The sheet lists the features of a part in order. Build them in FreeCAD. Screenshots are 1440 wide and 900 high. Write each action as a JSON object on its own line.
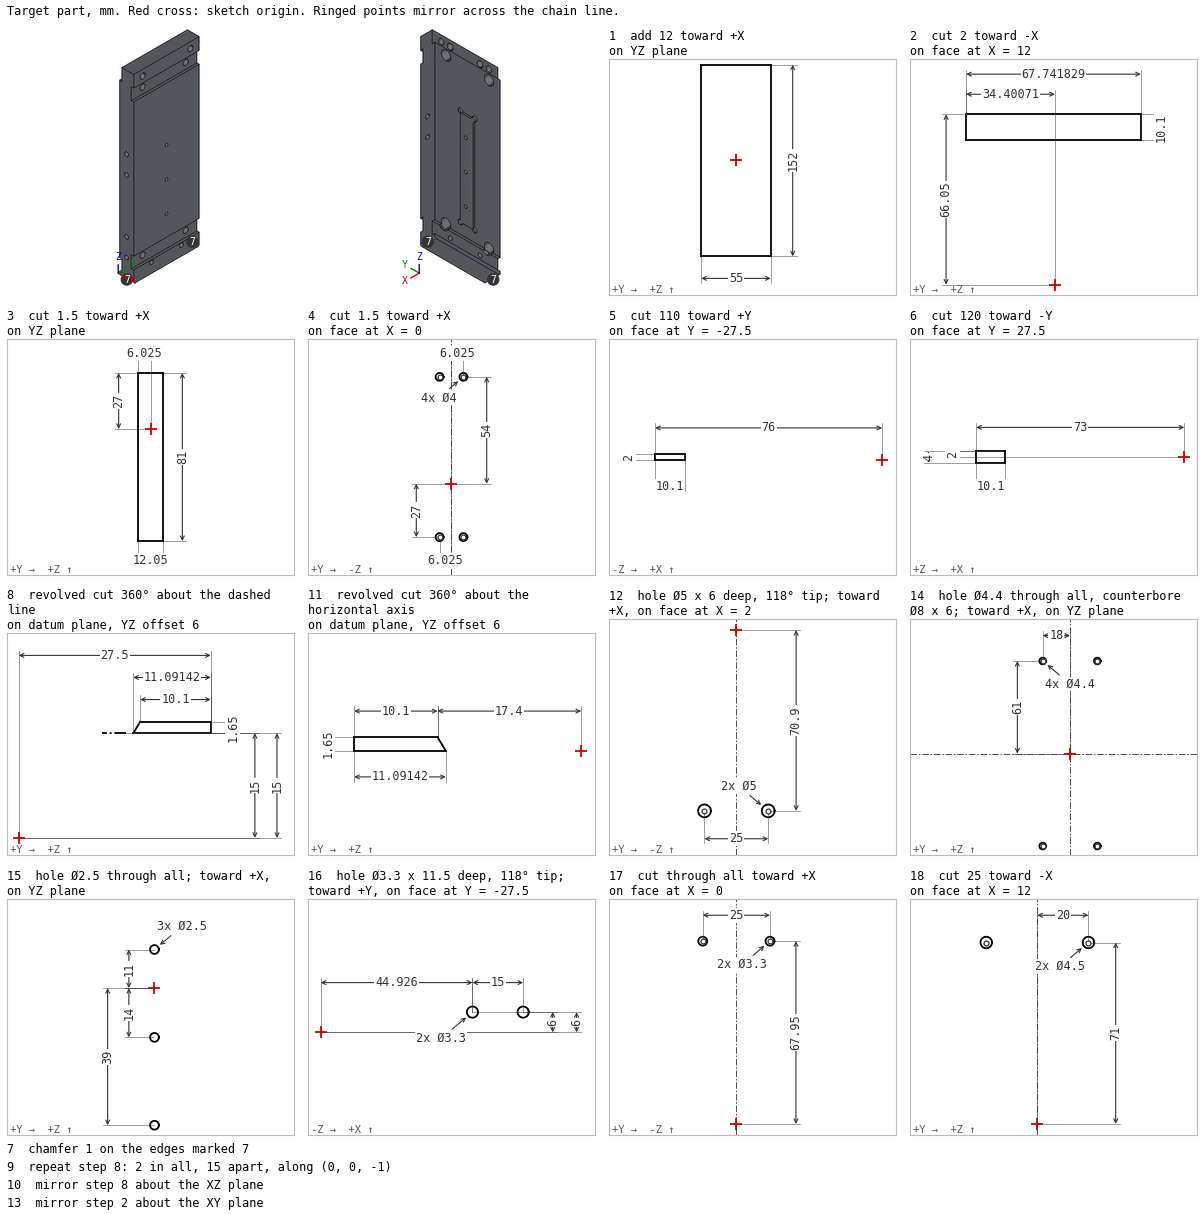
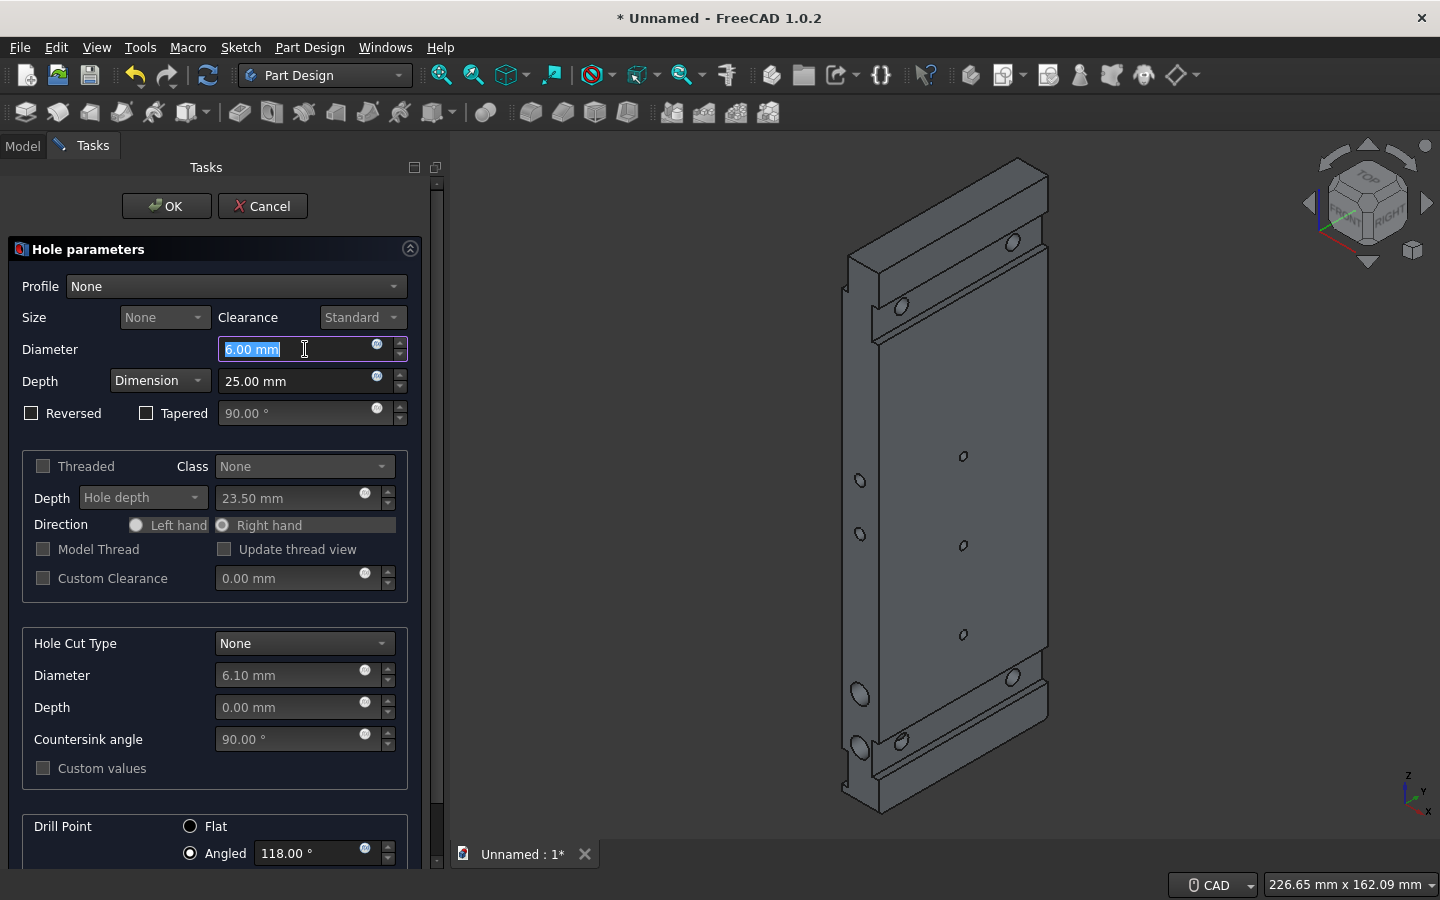
{"action": "type", "text": "3.3"}
{"action": "key", "text": "Tab"}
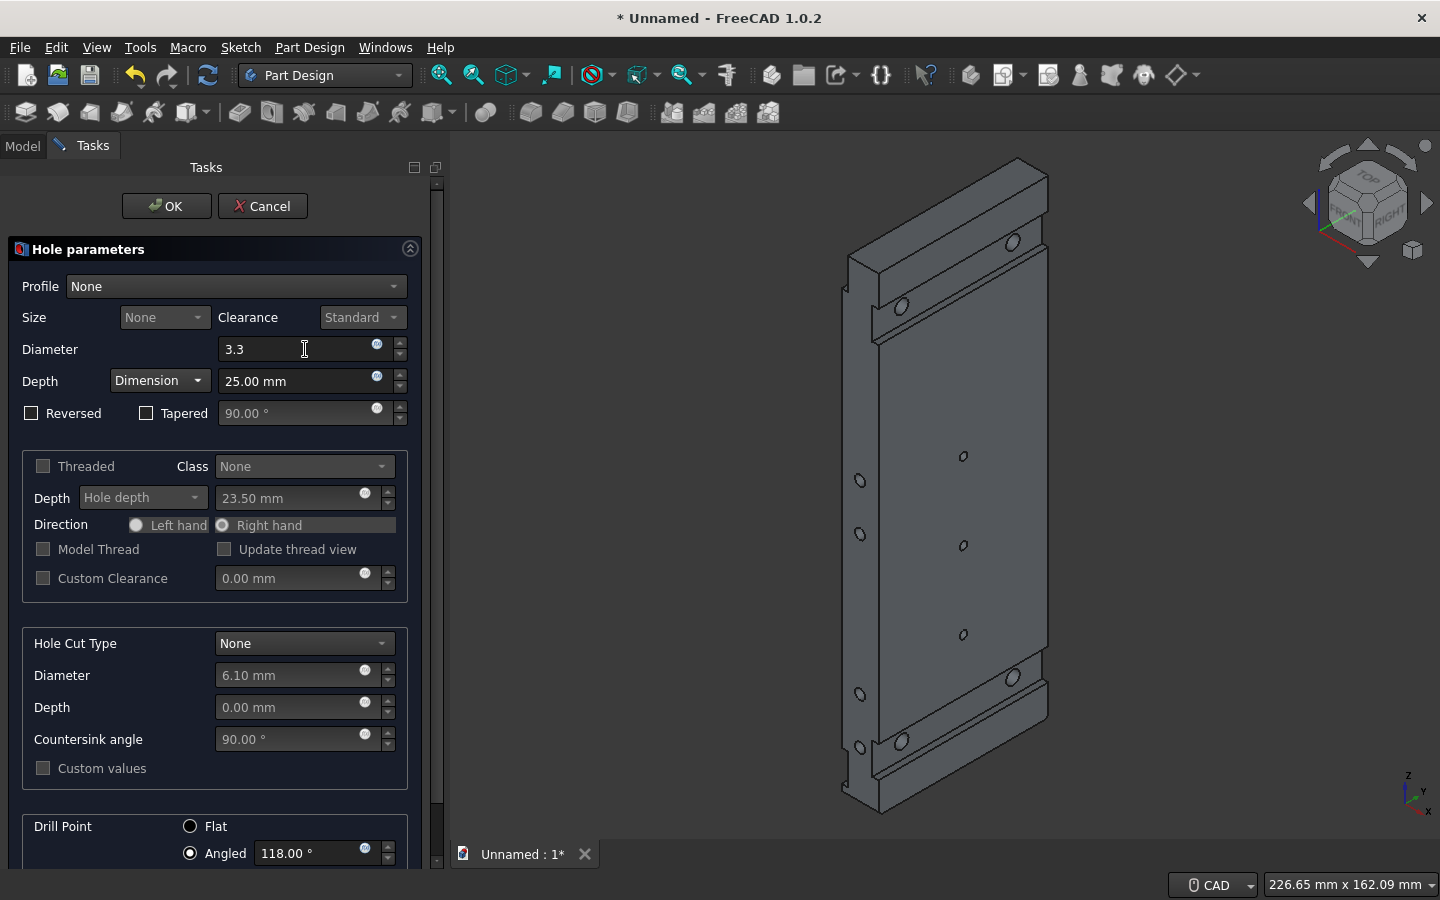
{"action": "triple_click", "coordinate": [305, 381]}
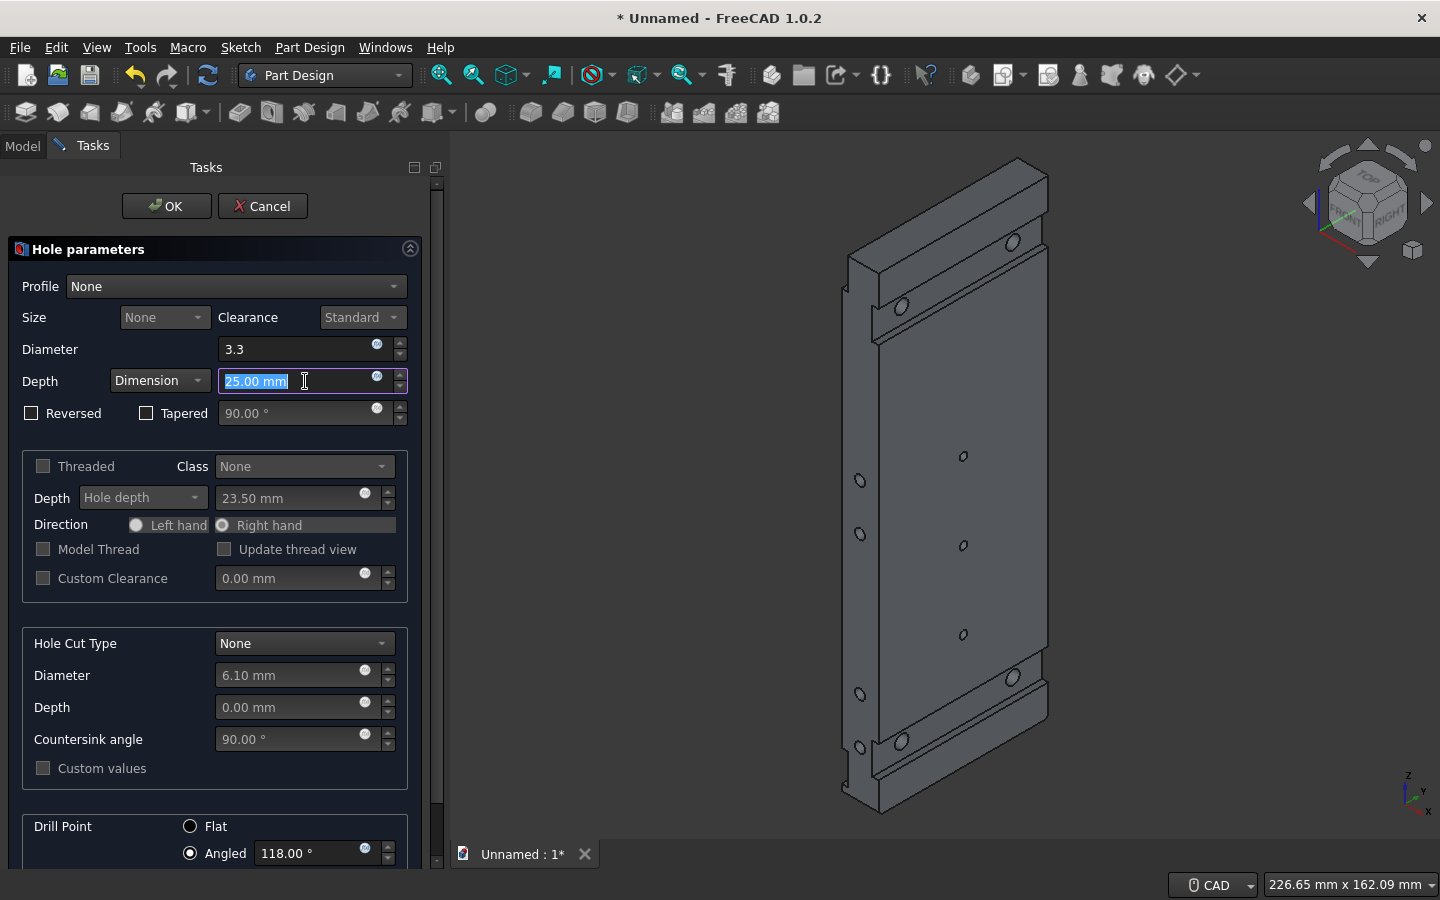
{"action": "type", "text": "11.5"}
{"action": "key", "text": "Tab"}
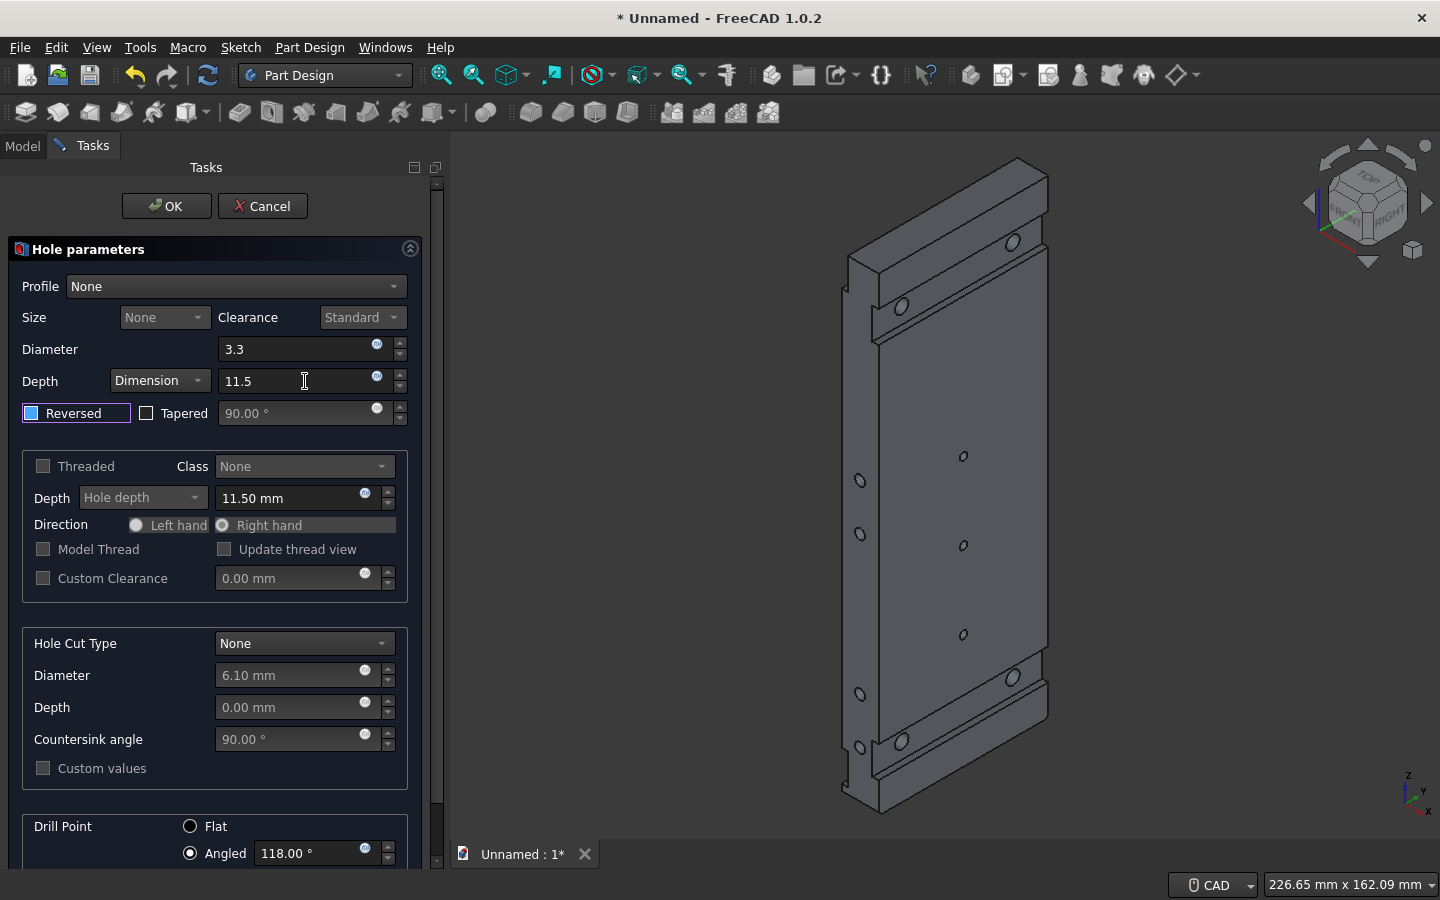
{"action": "left_click", "coordinate": [167, 206]}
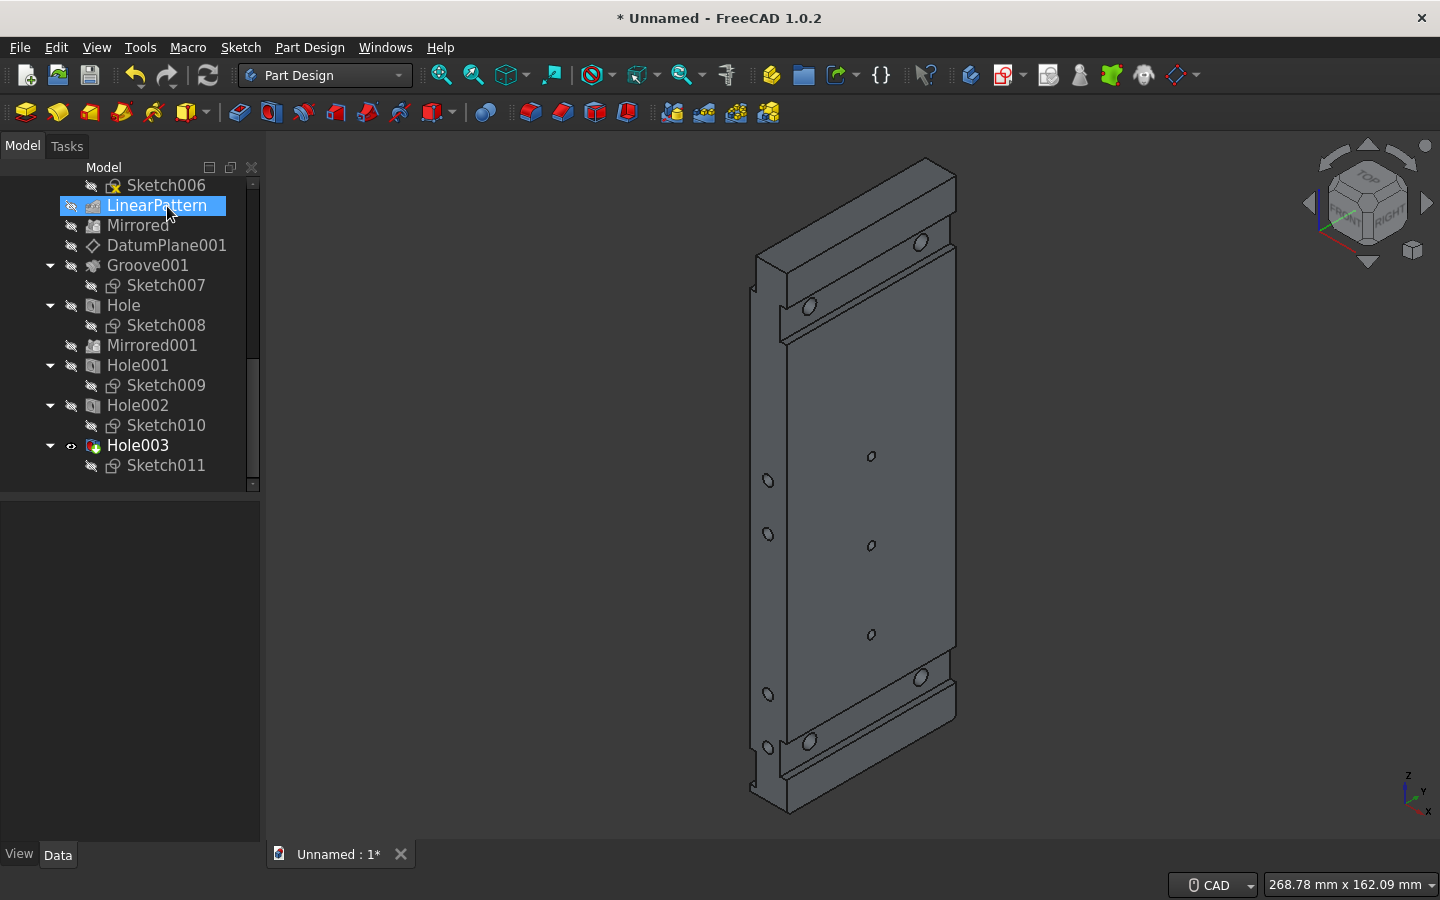
{"action": "key", "text": "6"}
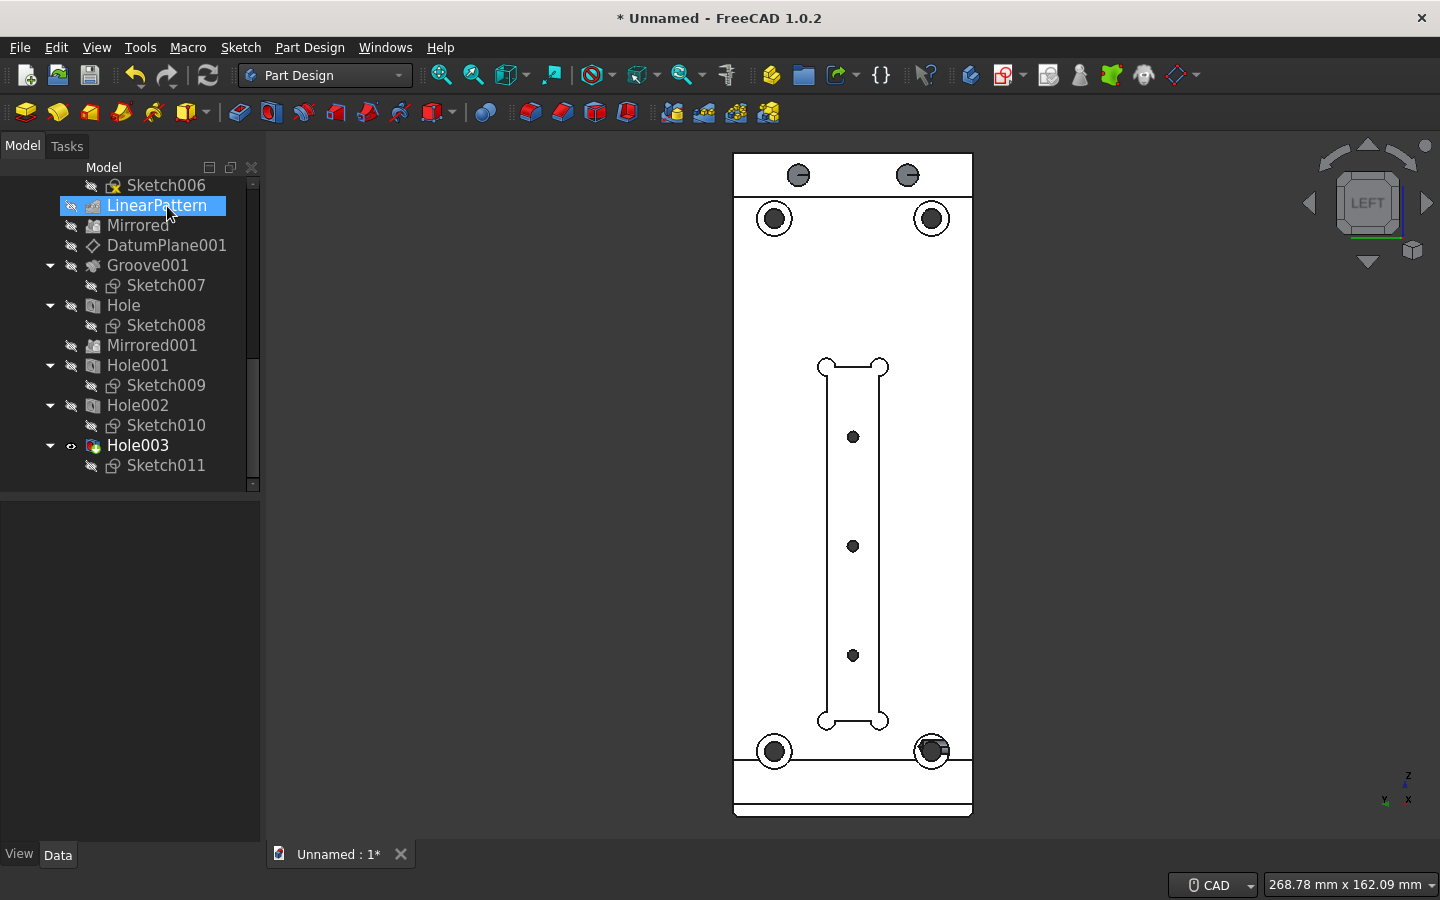
{"action": "left_click", "coordinate": [784, 317]}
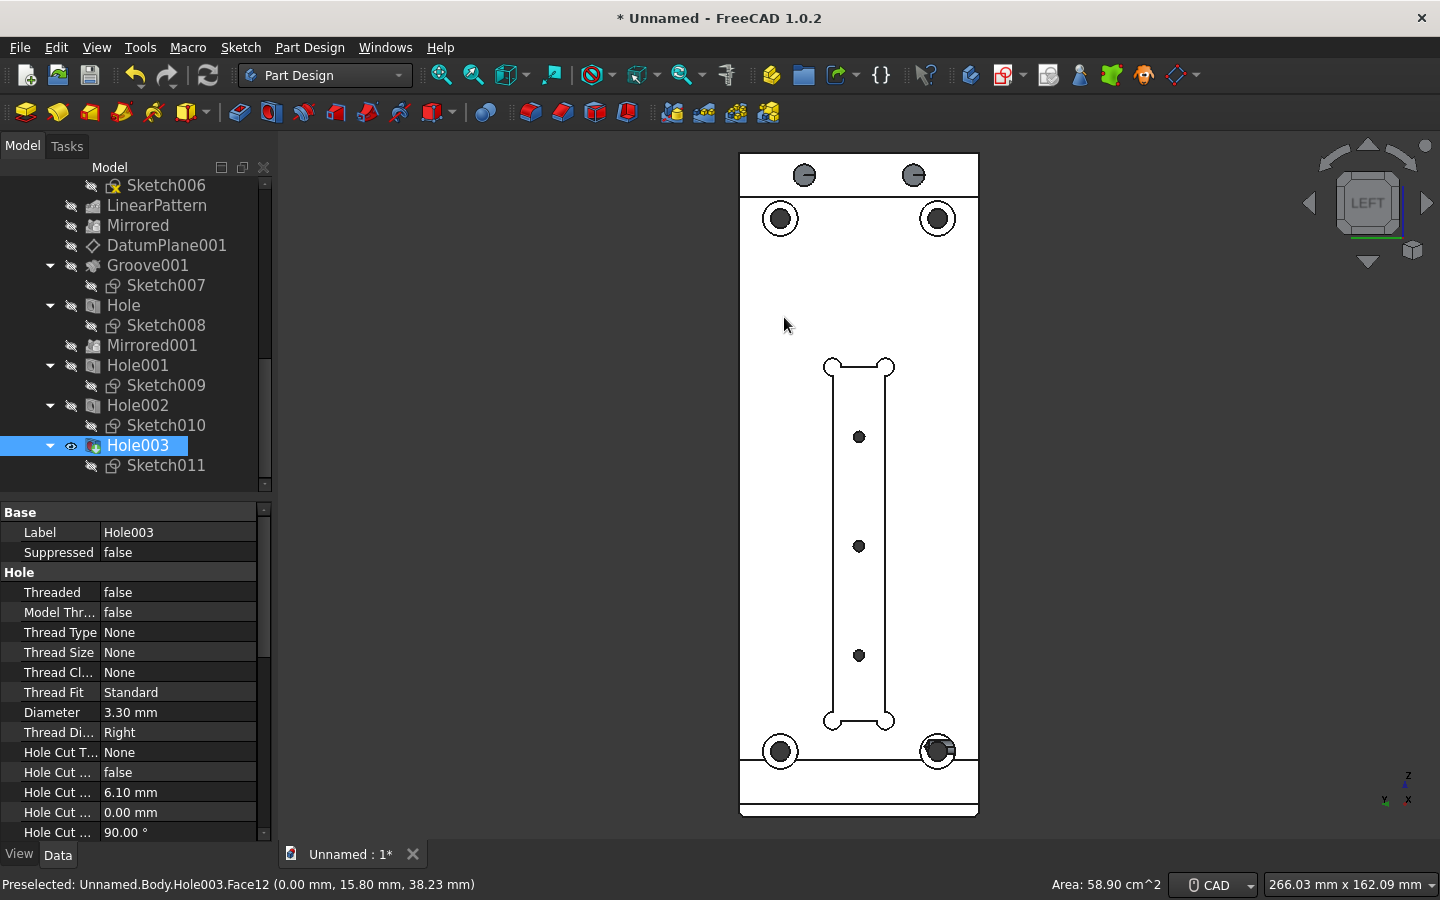
{"action": "left_click", "coordinate": [1004, 76]}